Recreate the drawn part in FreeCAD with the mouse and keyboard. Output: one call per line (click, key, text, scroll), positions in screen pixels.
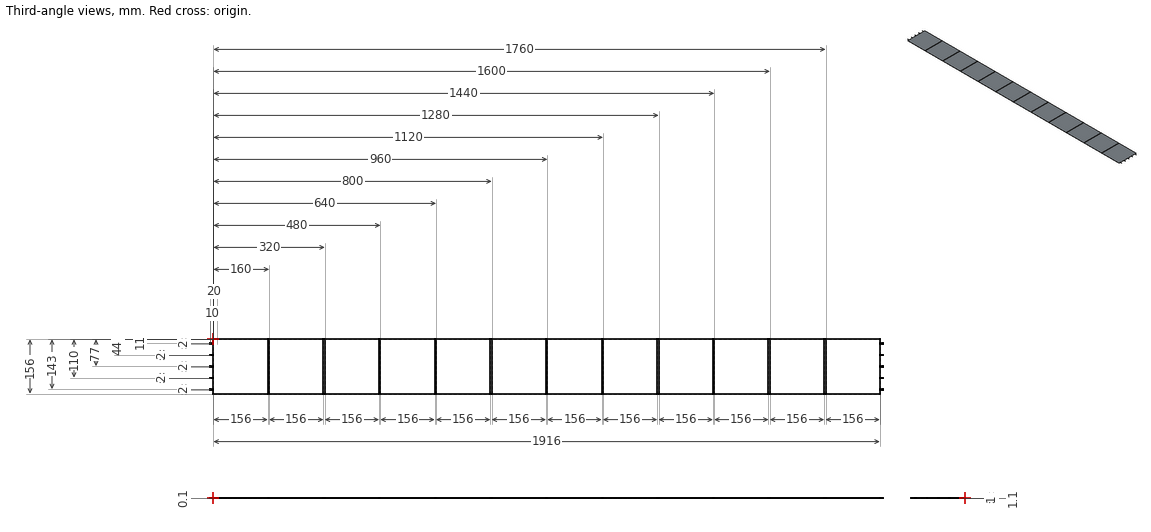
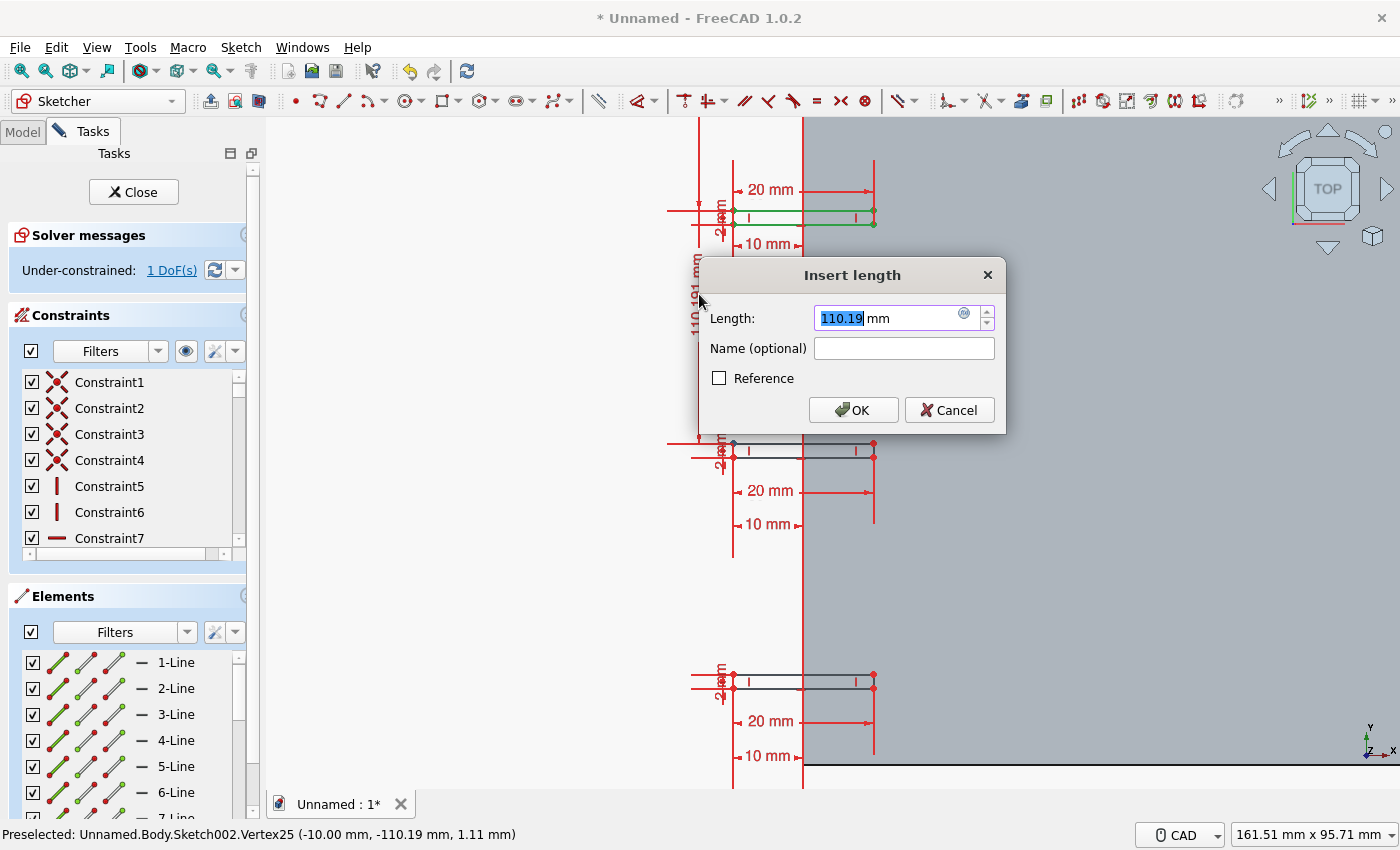
text(110)
key(Return)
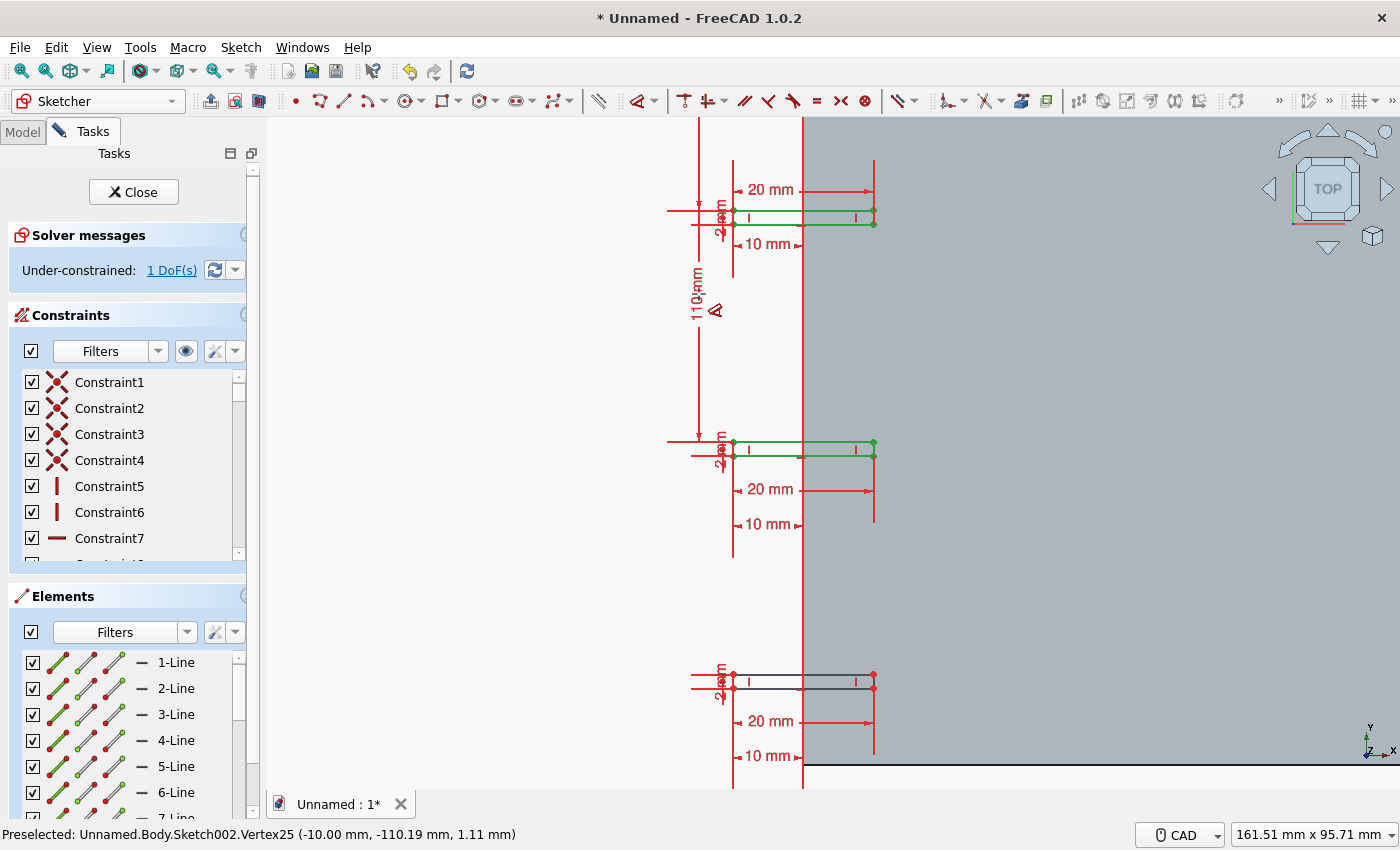
click(733, 675)
click(699, 410)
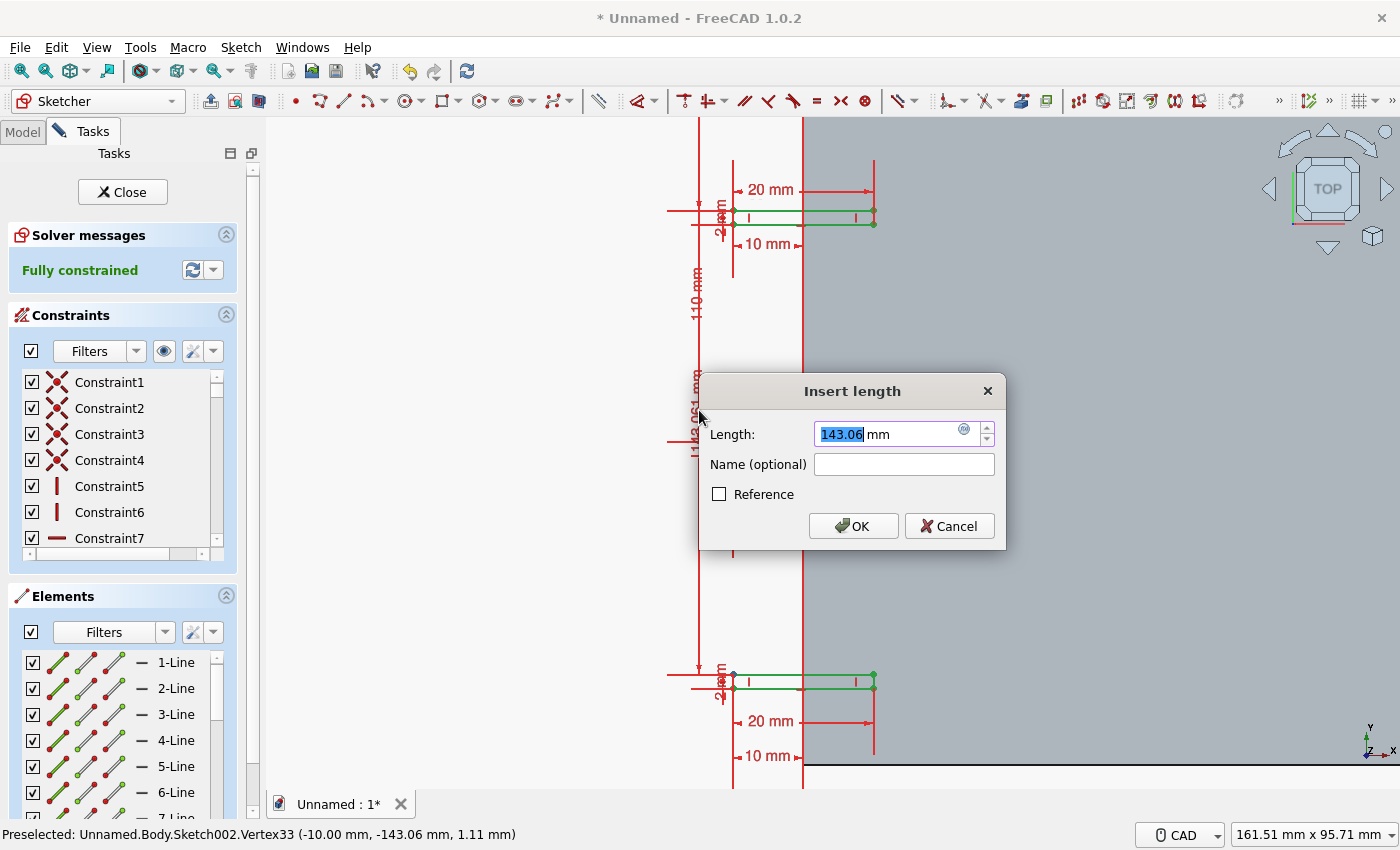
text(143)
key(Return)
key(Escape)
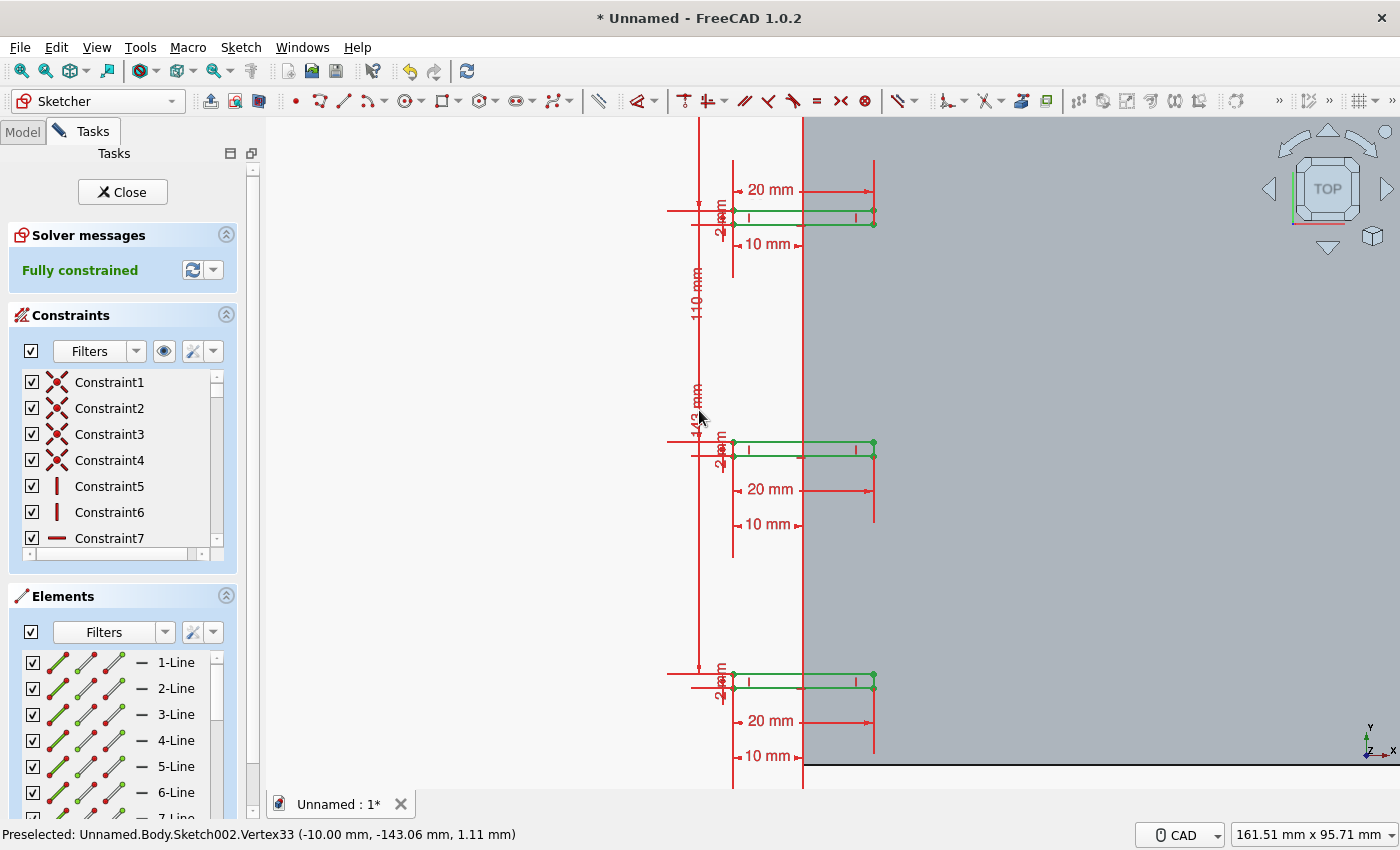
click(123, 192)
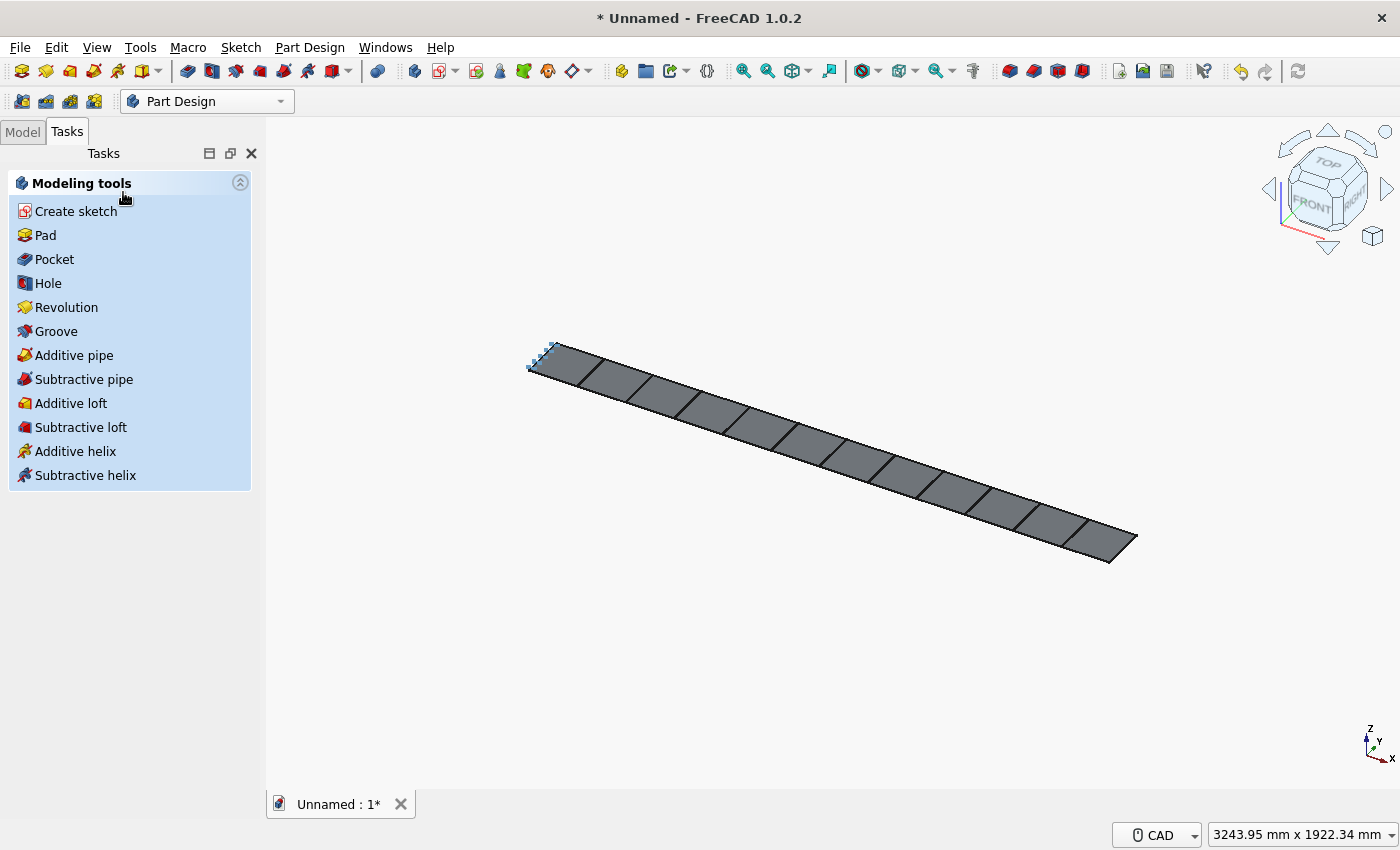
click(22, 72)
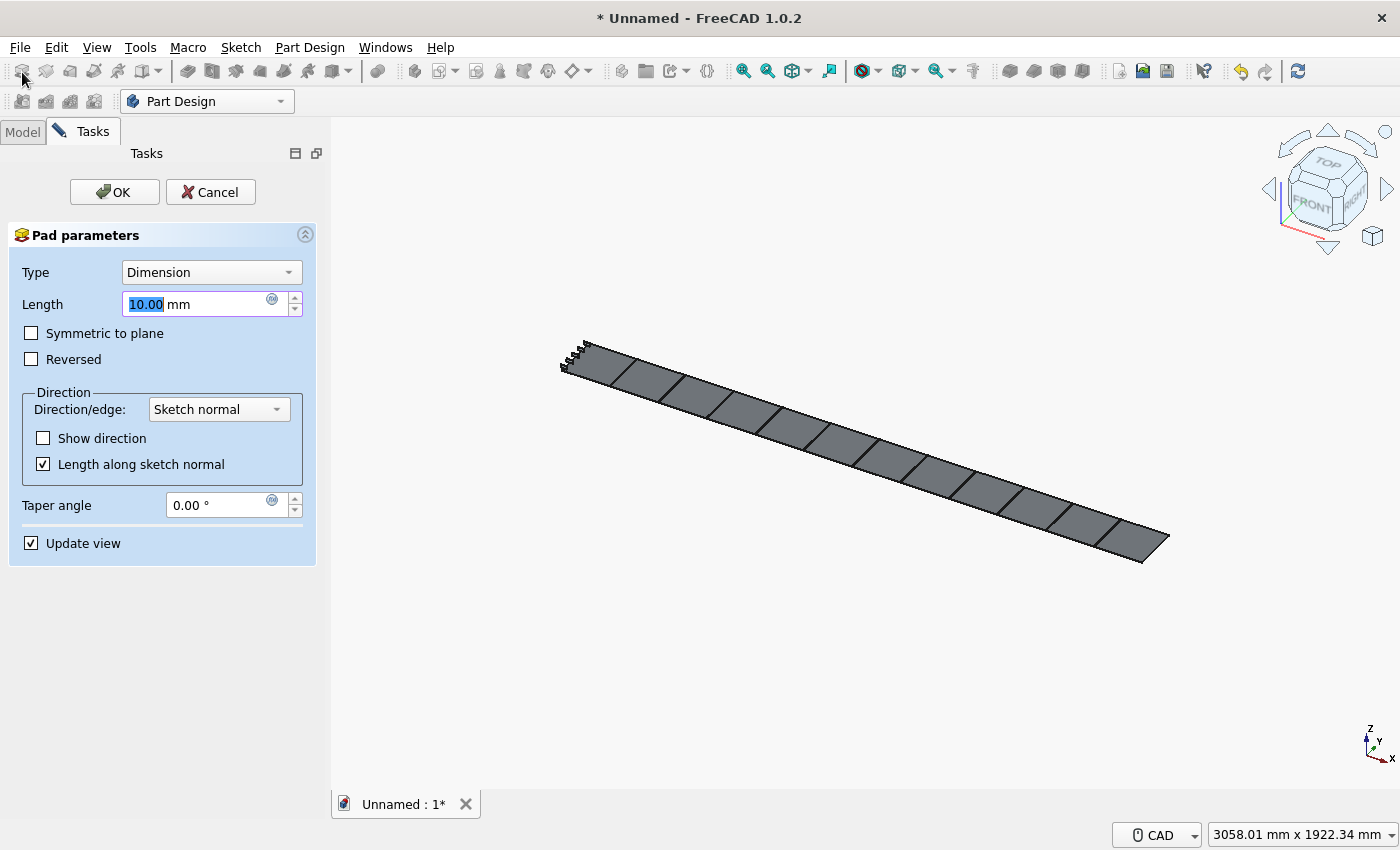
text(1.1)
key(Tab)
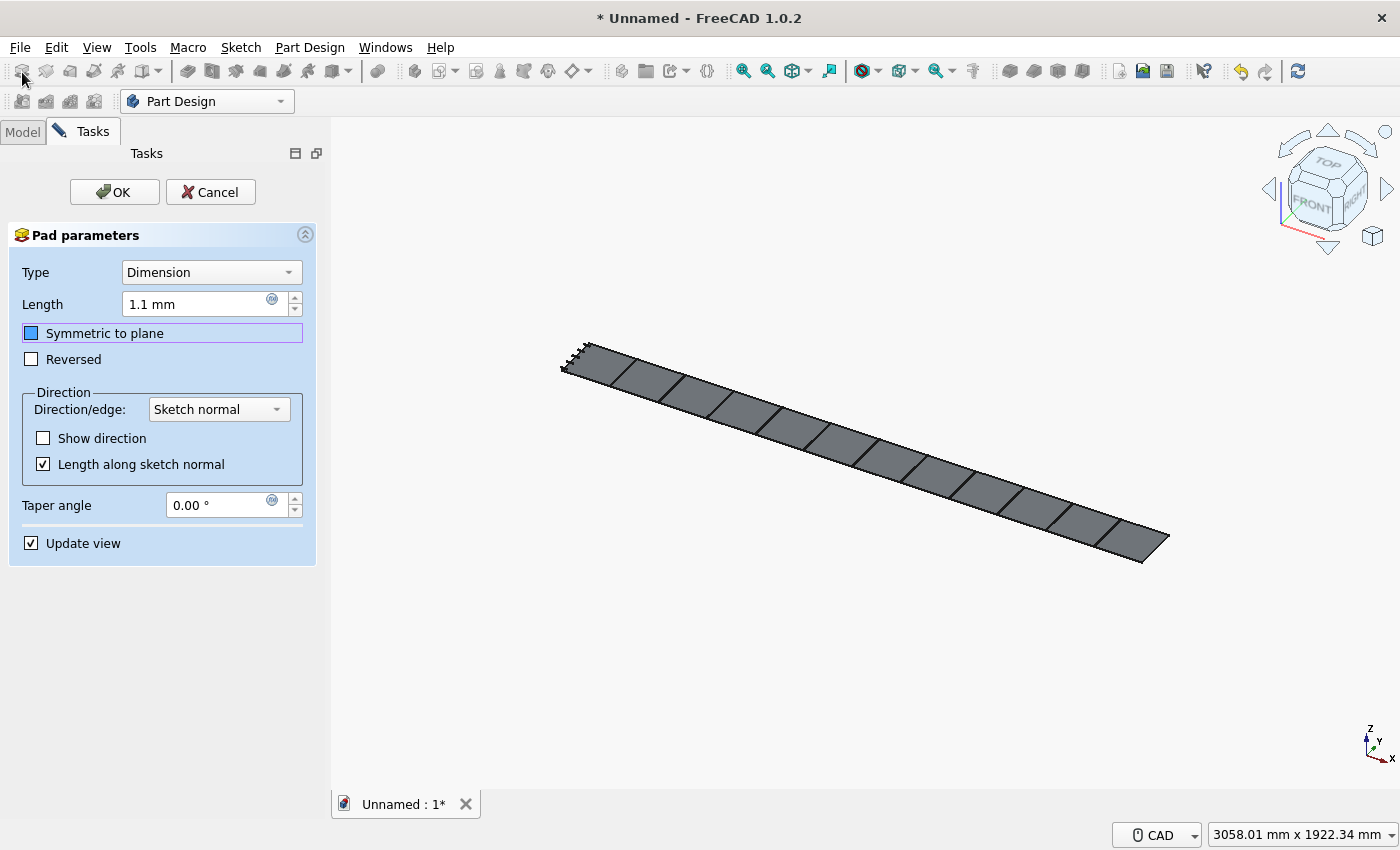
click(30, 359)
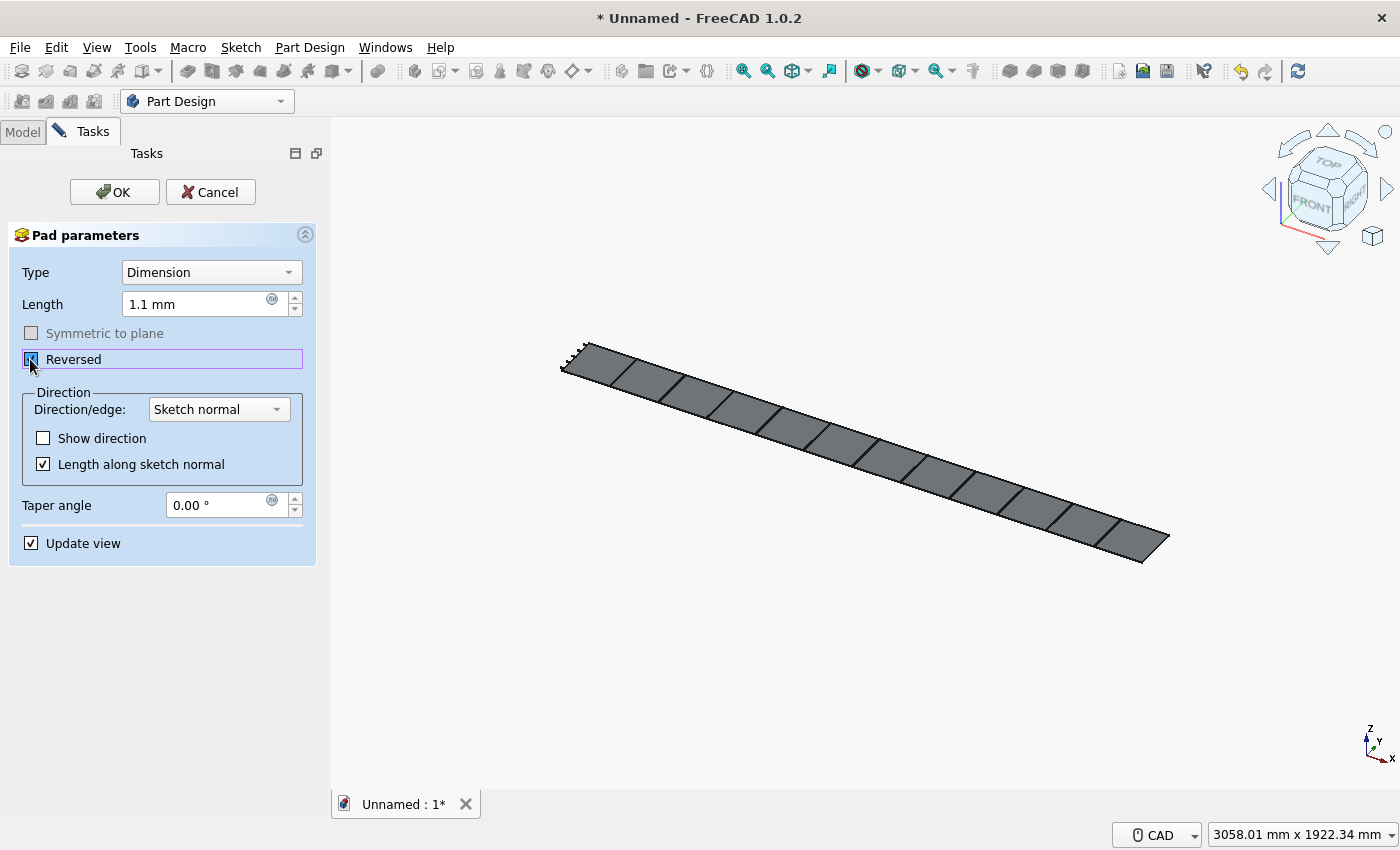
click(115, 192)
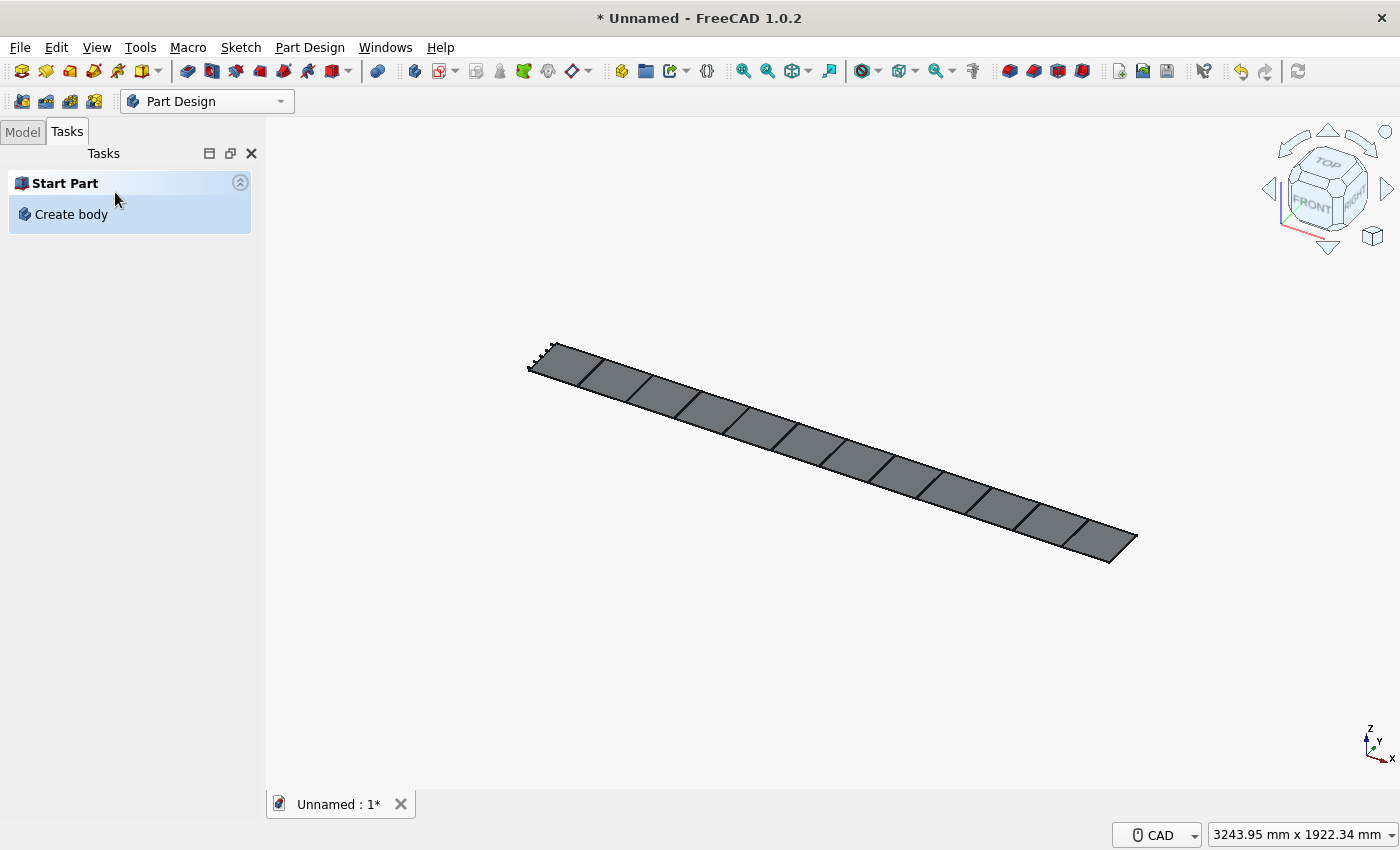
click(23, 131)